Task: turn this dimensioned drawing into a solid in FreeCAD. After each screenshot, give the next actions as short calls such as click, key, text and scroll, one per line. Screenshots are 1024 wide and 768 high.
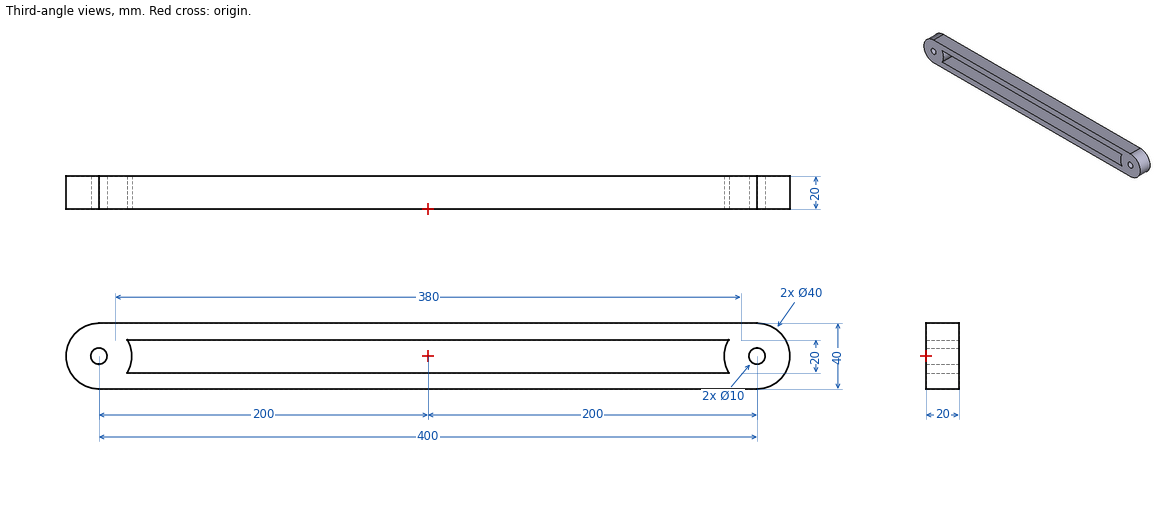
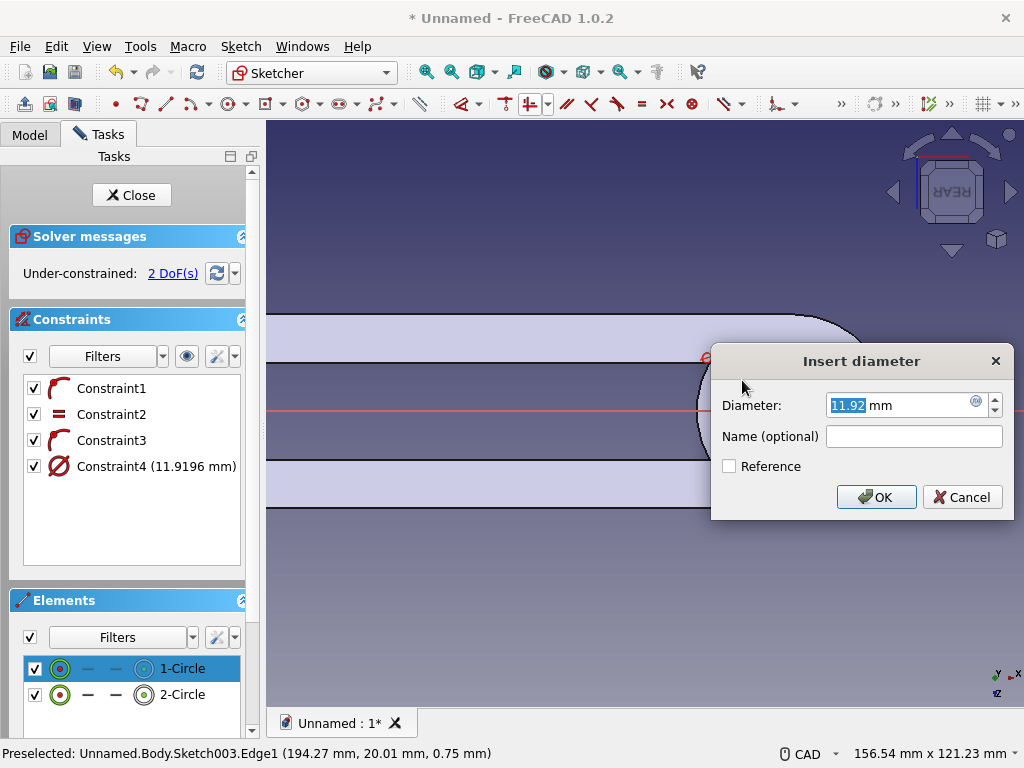
text(10)
key(Return)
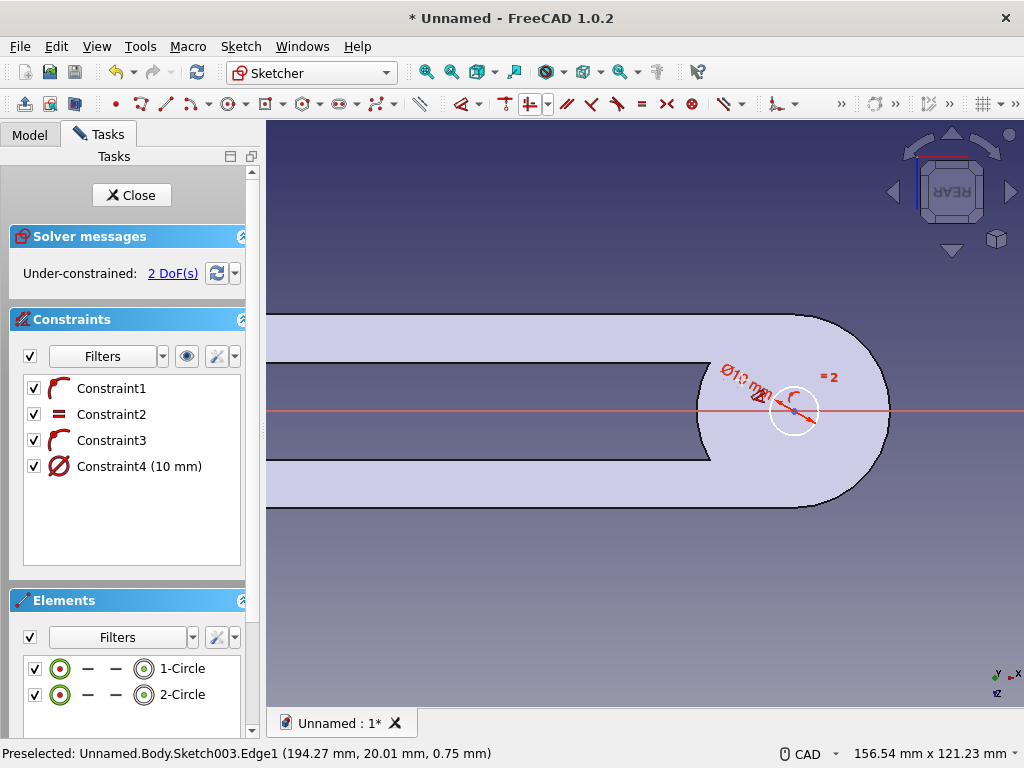
scroll(767, 414, down, 8)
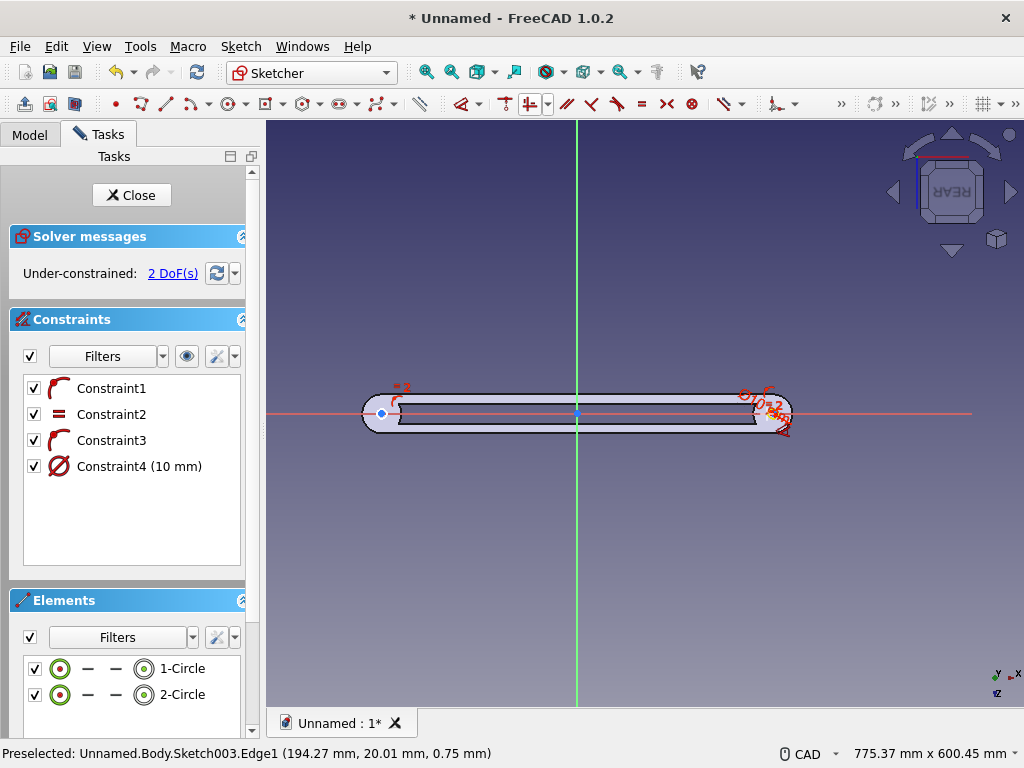
click(773, 414)
click(675, 448)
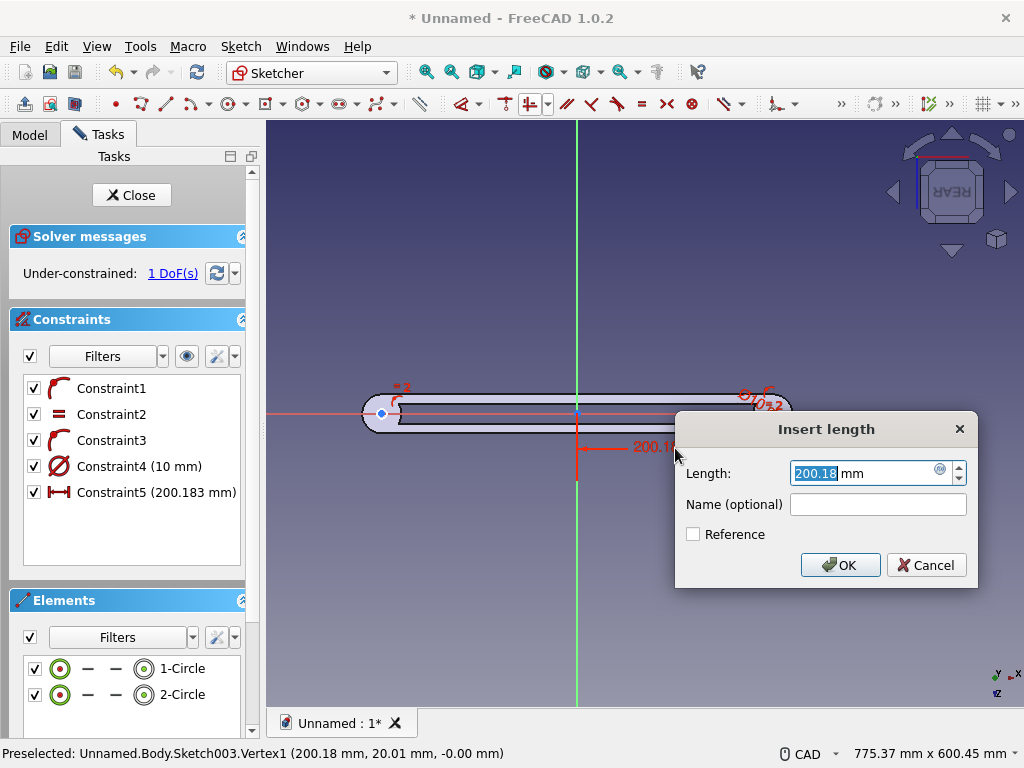
text(200)
key(Return)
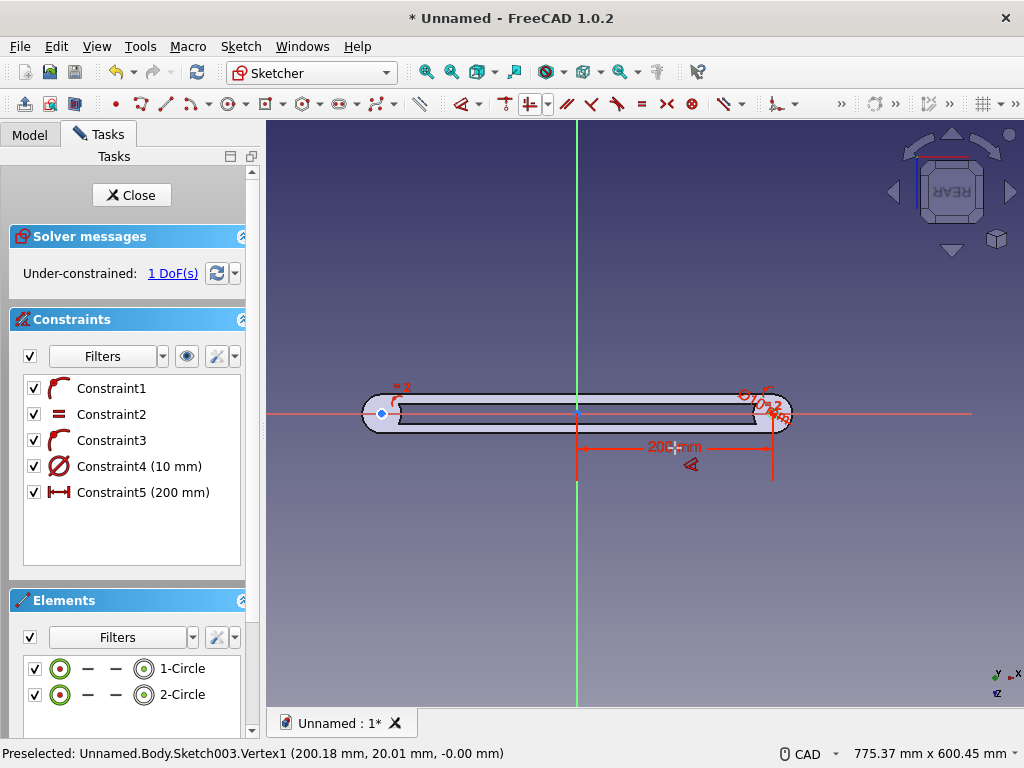
click(382, 414)
click(480, 448)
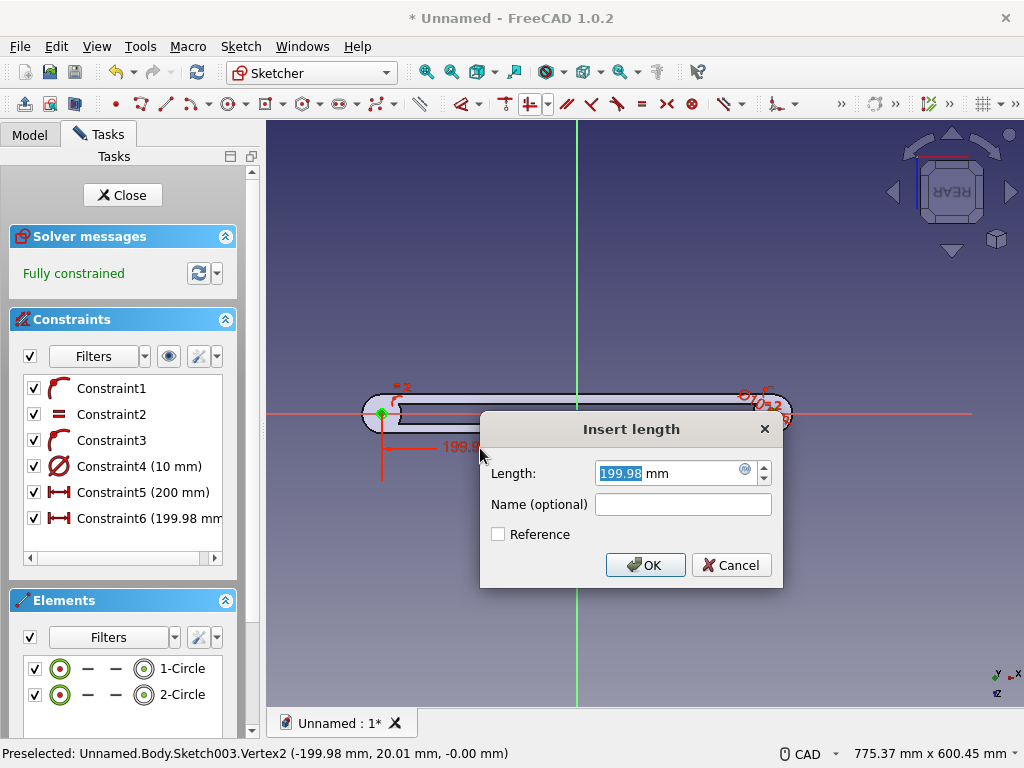
text(200)
key(Return)
key(Escape)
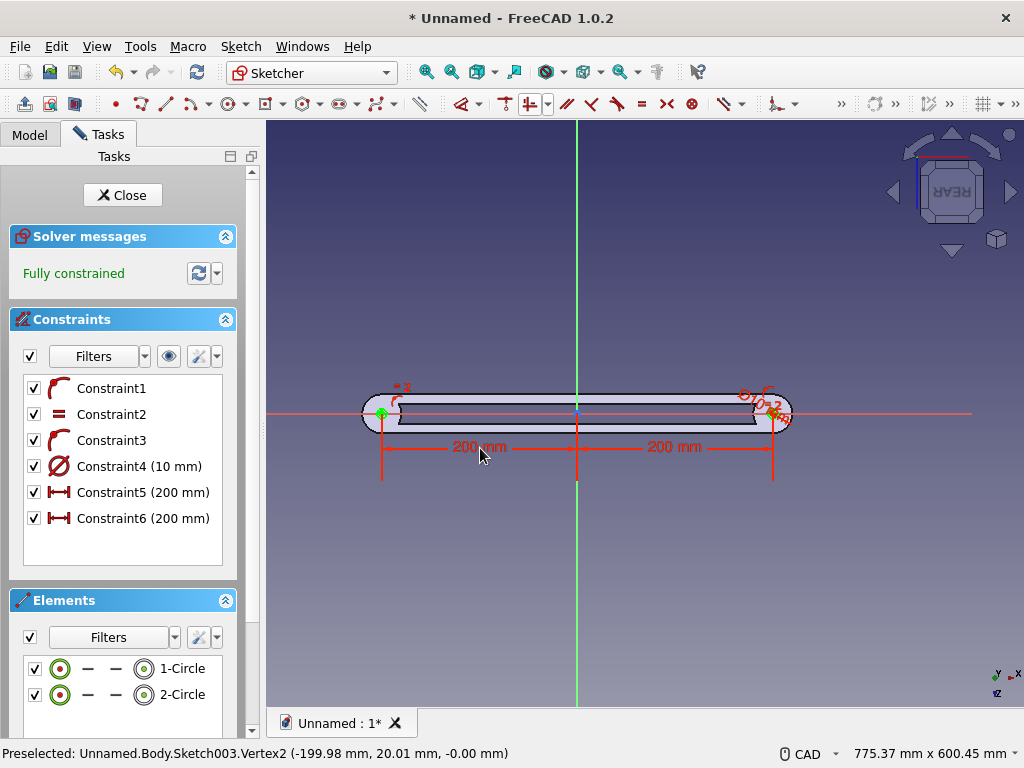
click(123, 195)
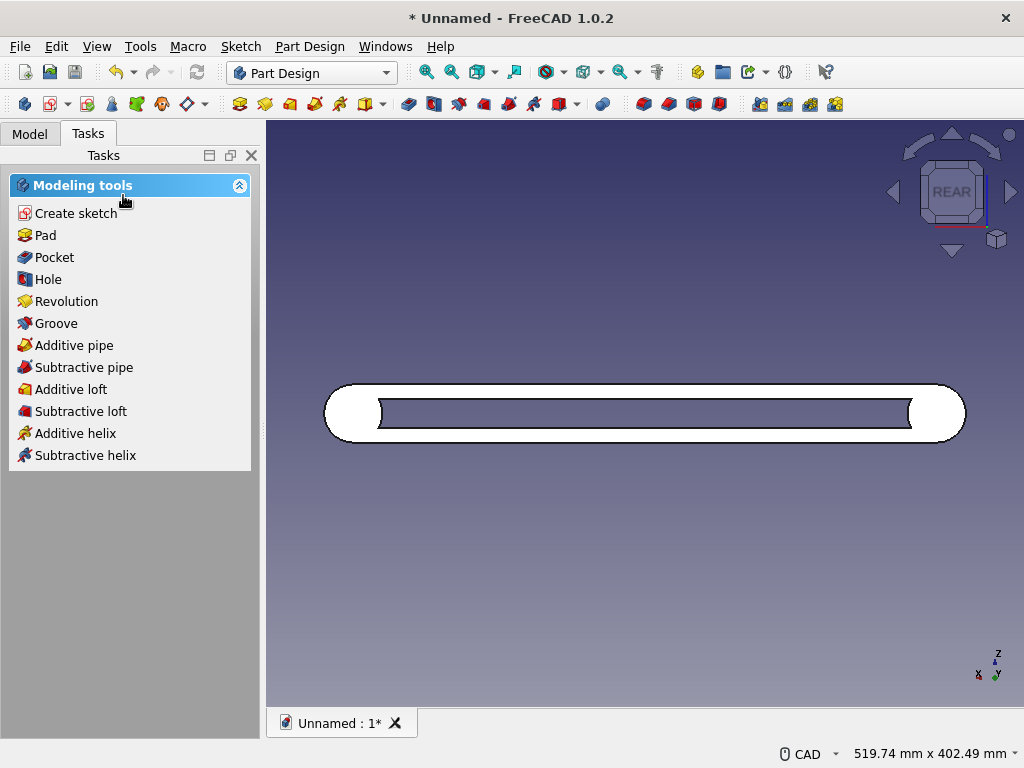
click(409, 104)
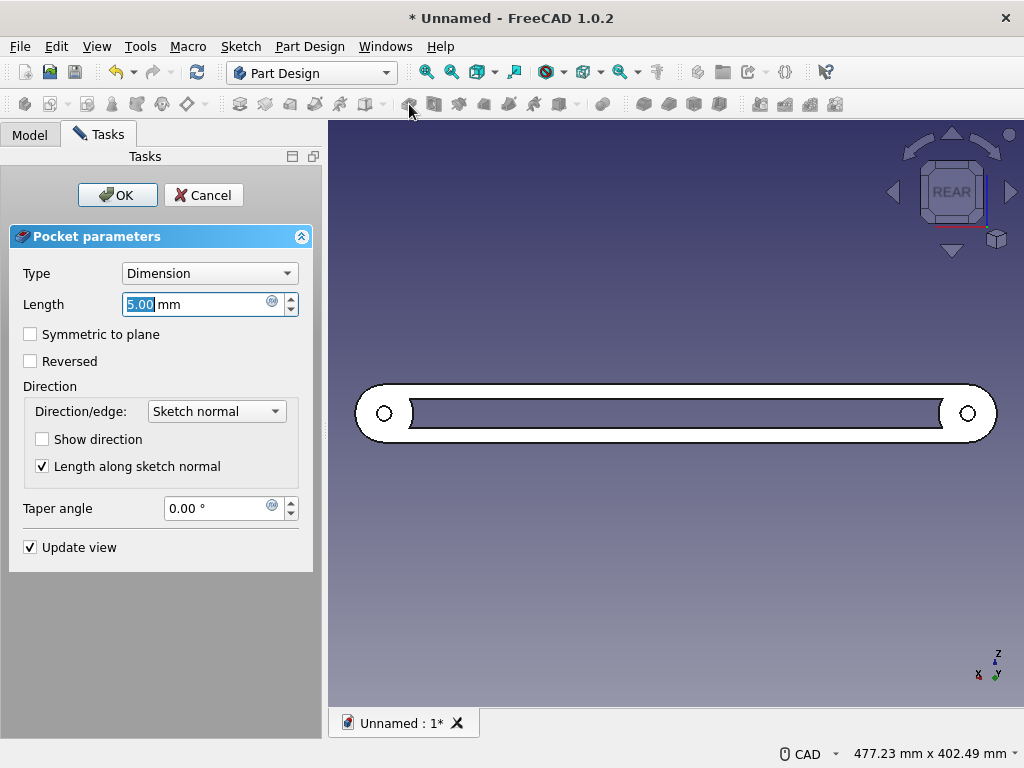
click(210, 274)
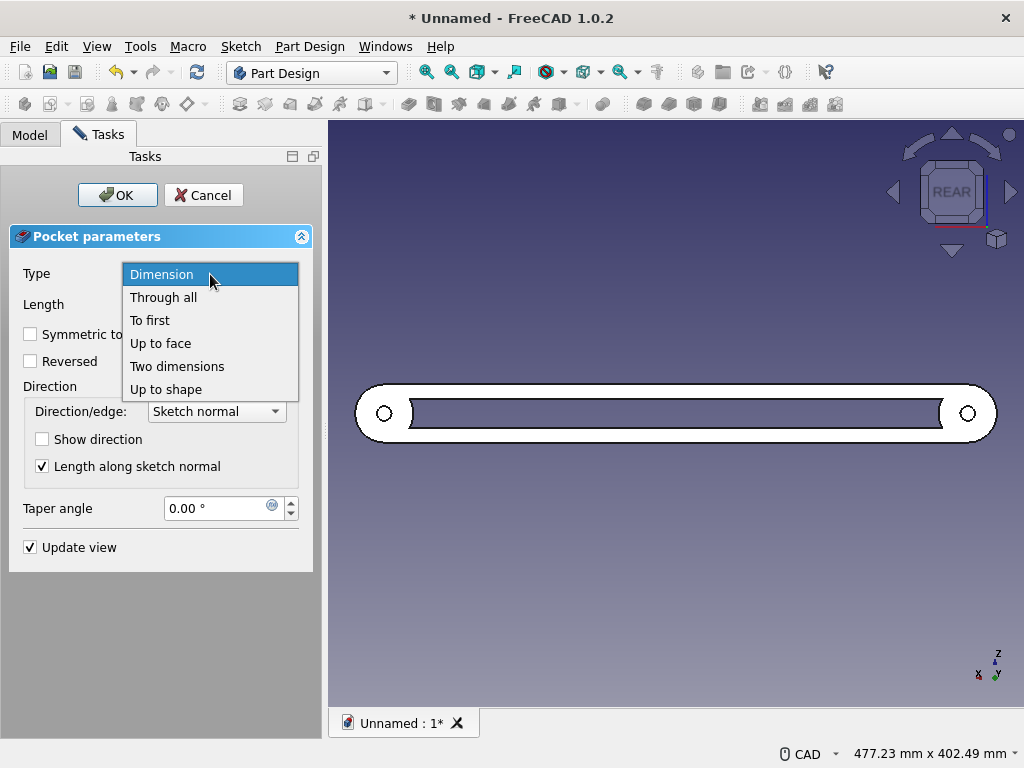
click(208, 298)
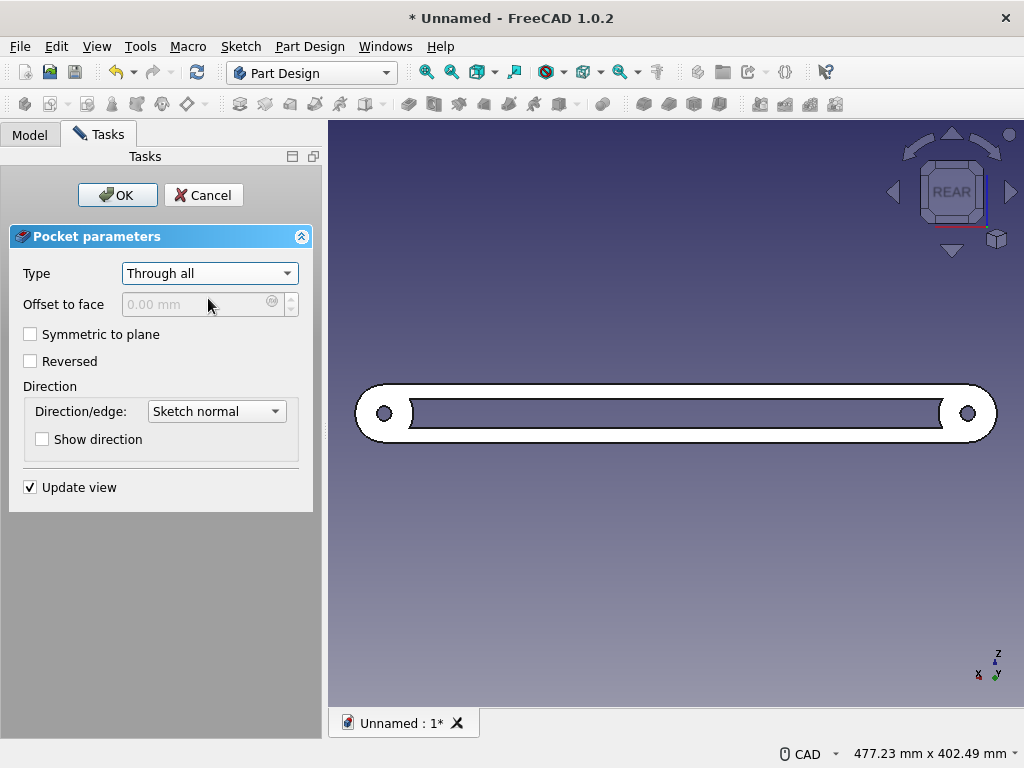
click(118, 195)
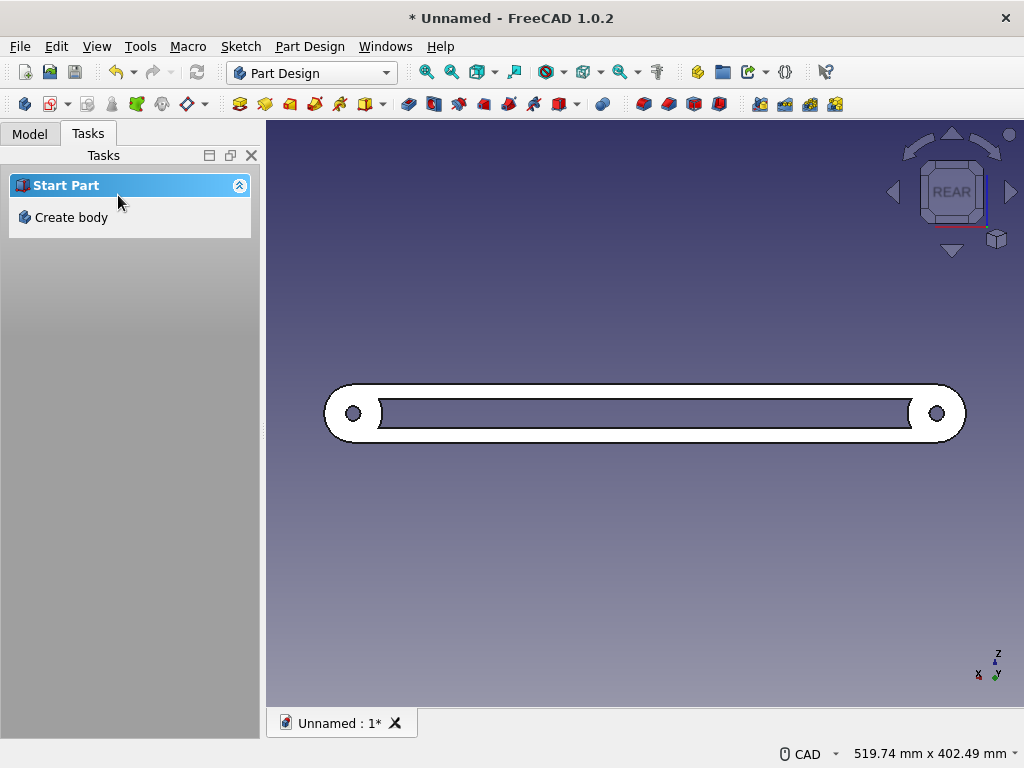
key(0)